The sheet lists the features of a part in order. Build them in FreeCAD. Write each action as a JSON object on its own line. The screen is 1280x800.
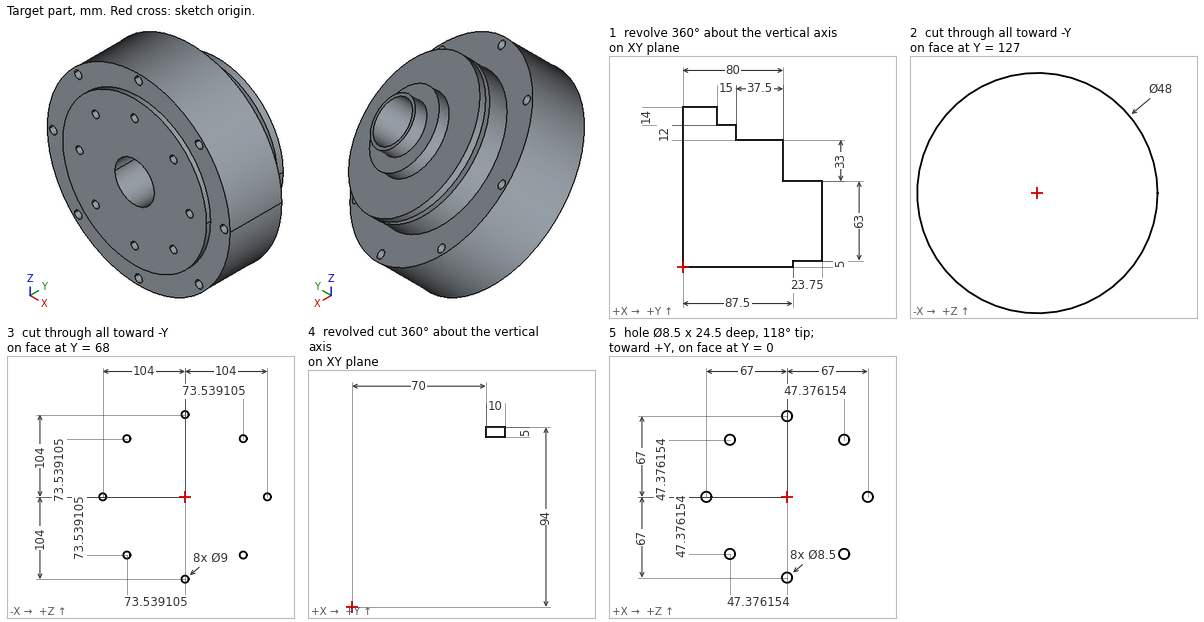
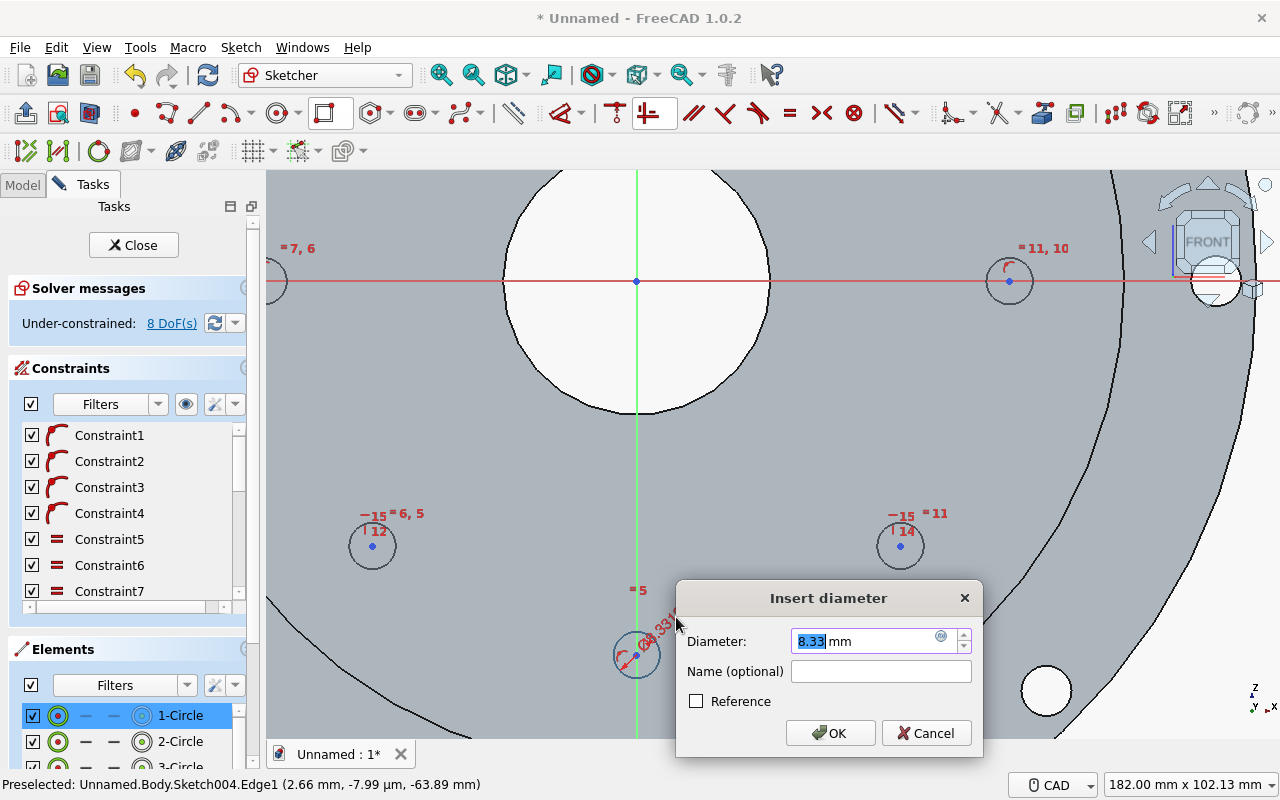
{"action": "type", "text": "8.5"}
{"action": "key", "text": "Return"}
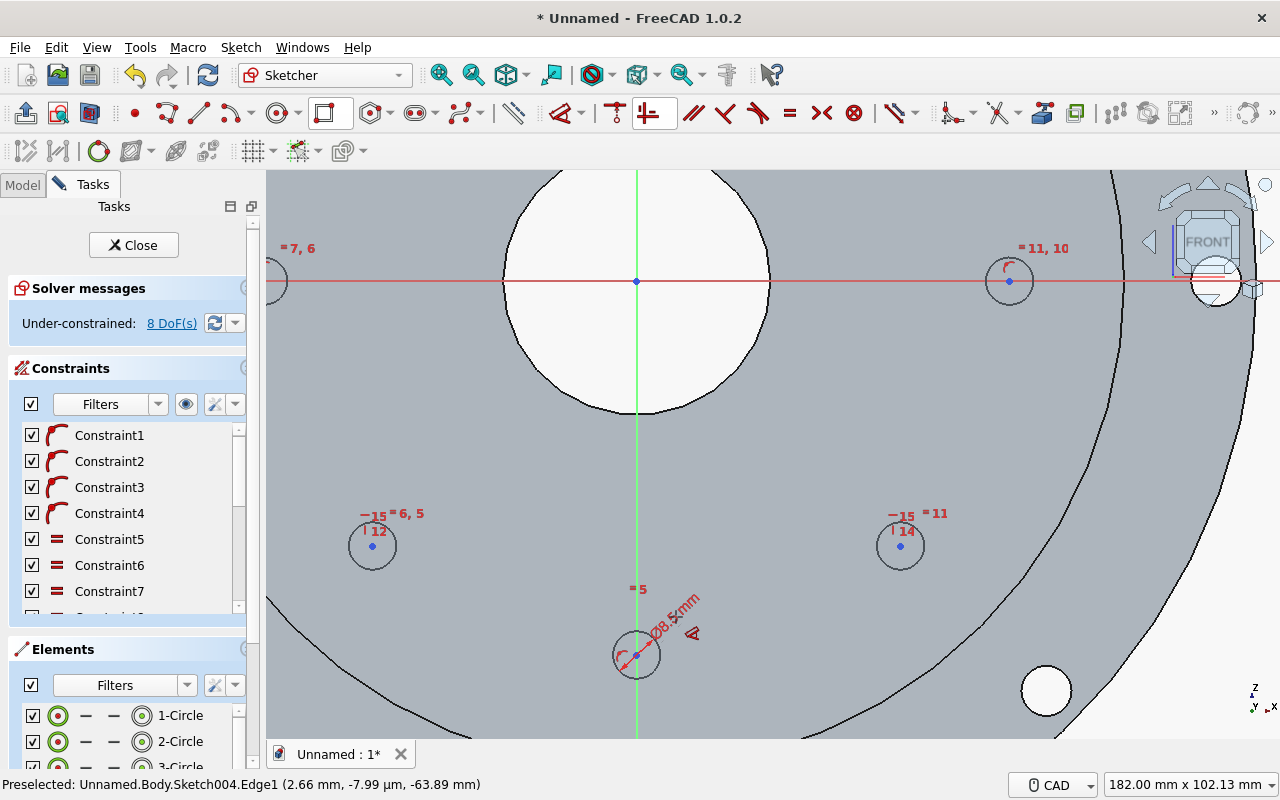
{"action": "left_click", "coordinate": [637, 655]}
{"action": "left_click", "coordinate": [671, 468]}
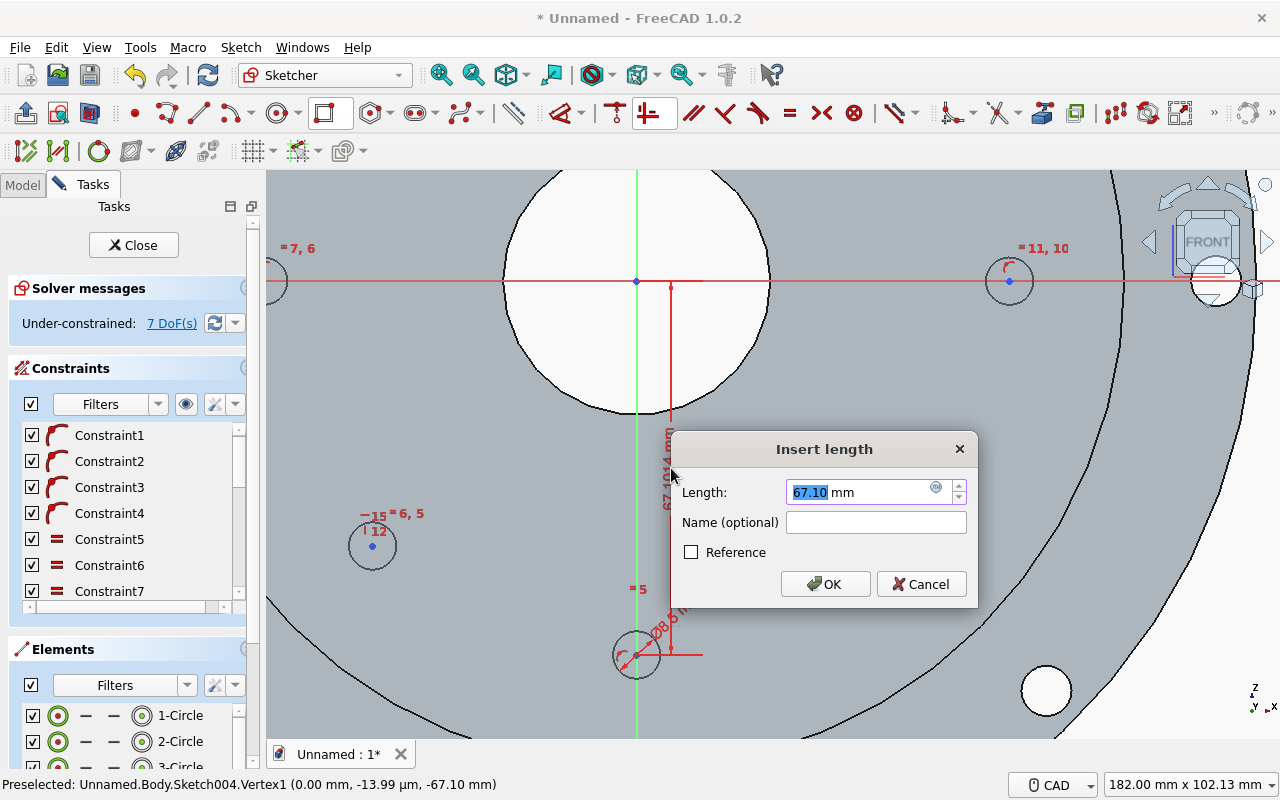
{"action": "type", "text": "67"}
{"action": "key", "text": "Return"}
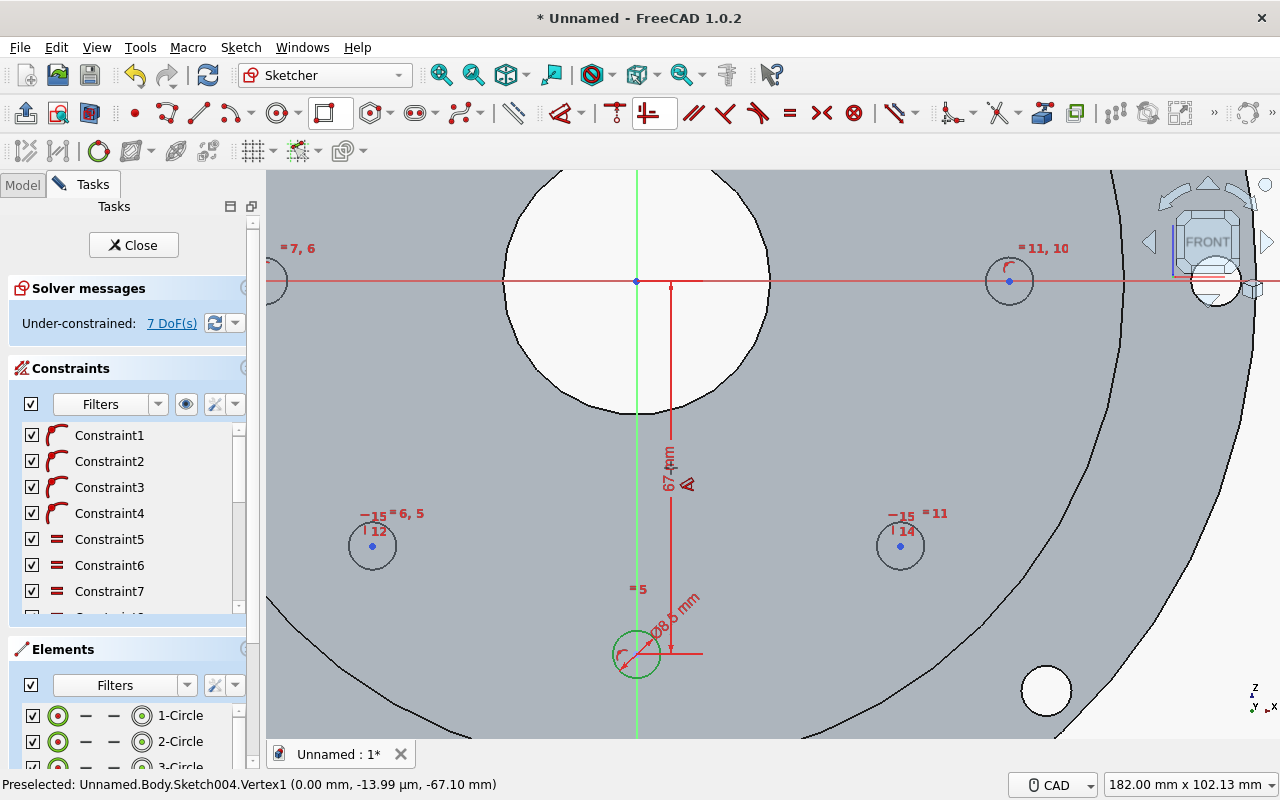
{"action": "scroll", "coordinate": [760, 596], "scroll_direction": "down", "scroll_amount": 4}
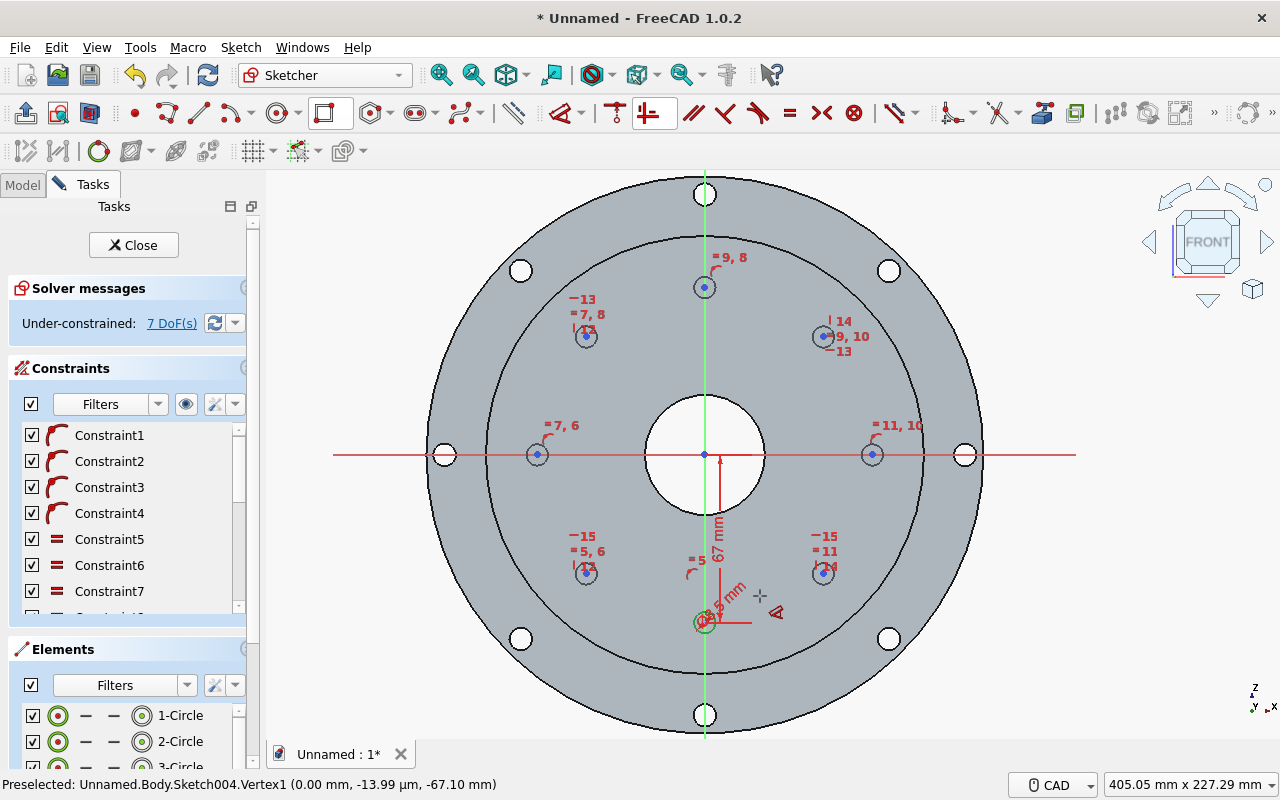
{"action": "left_click", "coordinate": [537, 455]}
{"action": "left_click", "coordinate": [621, 489]}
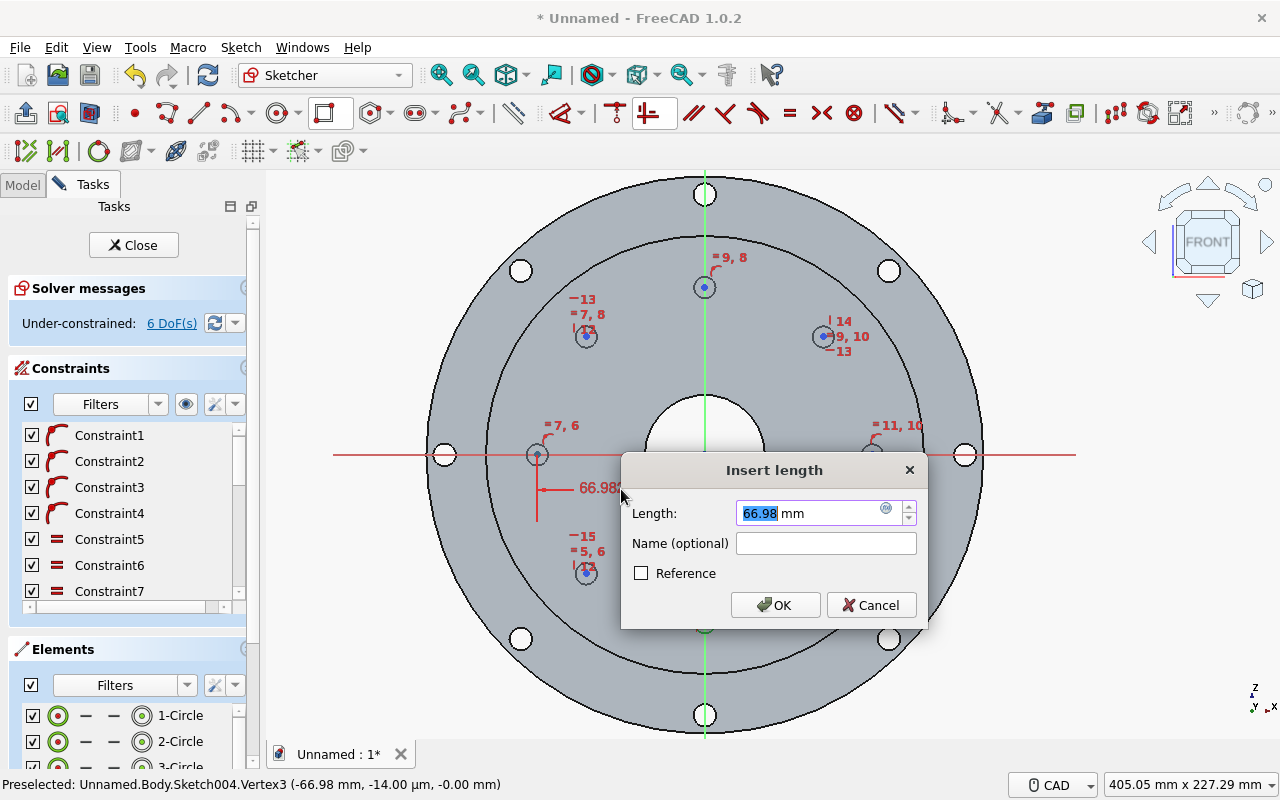
{"action": "type", "text": "67"}
{"action": "key", "text": "Return"}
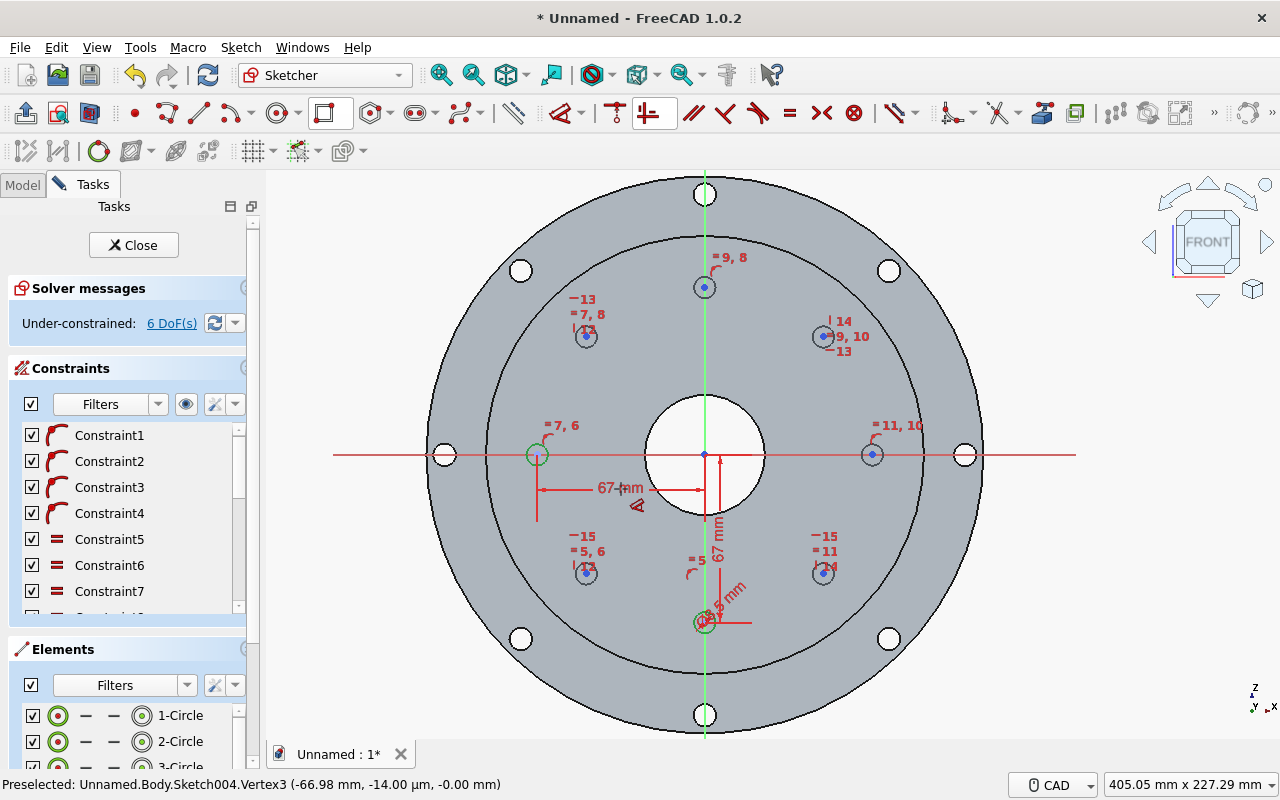
{"action": "left_click", "coordinate": [705, 288]}
{"action": "left_click", "coordinate": [739, 371]}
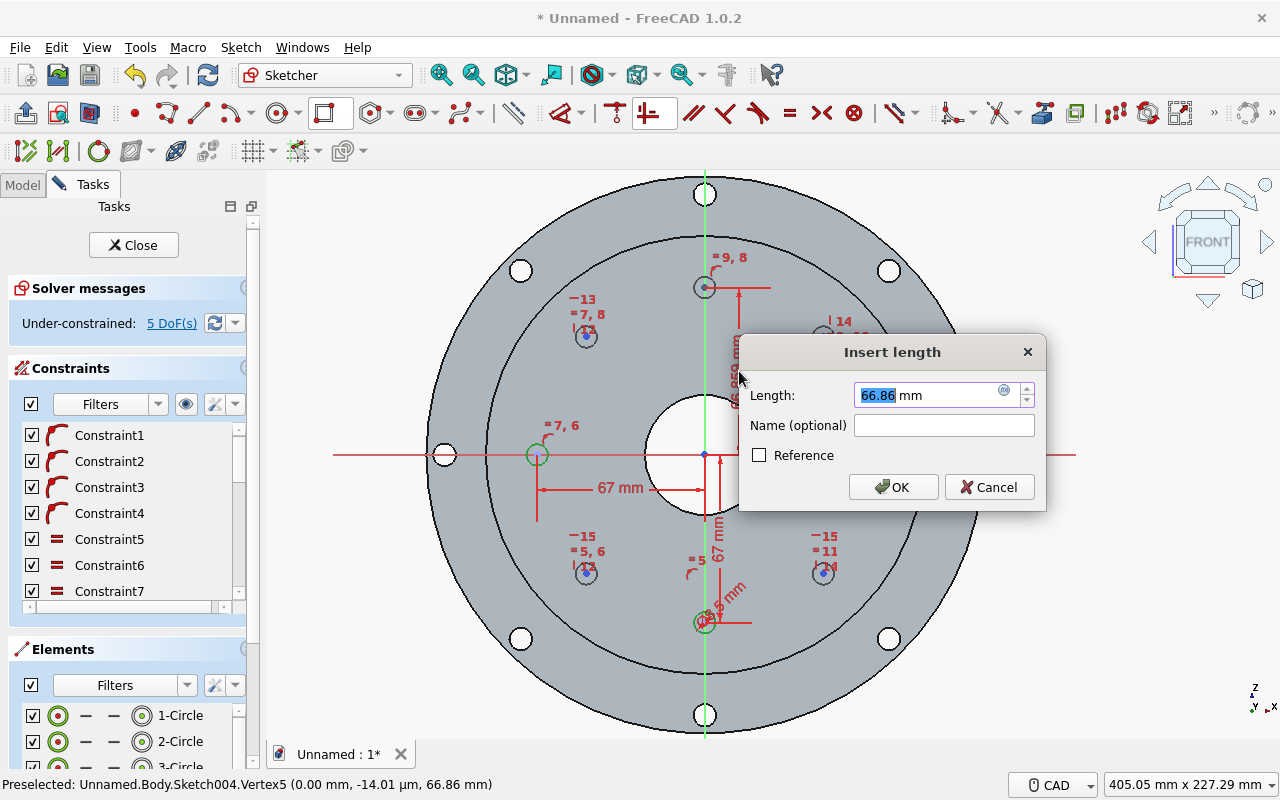
{"action": "type", "text": "67"}
{"action": "key", "text": "Return"}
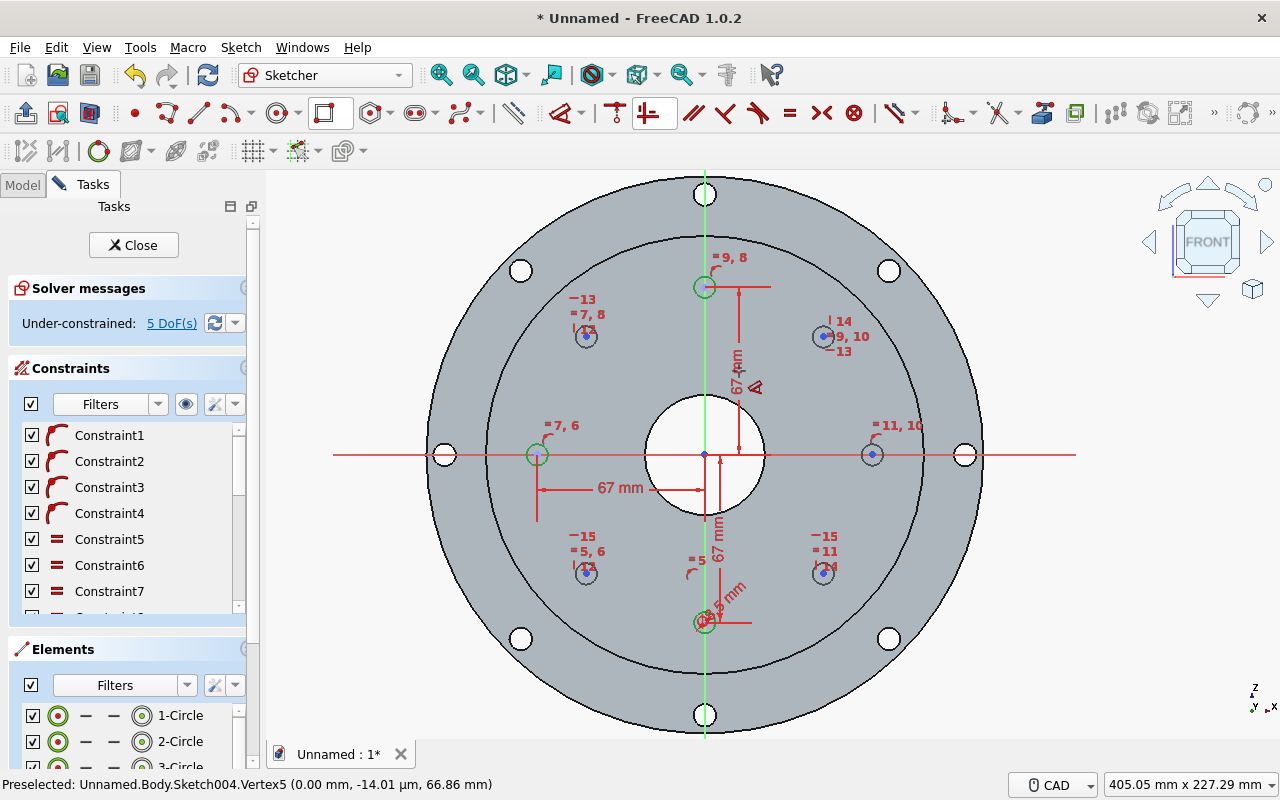
{"action": "left_click", "coordinate": [872, 455]}
{"action": "left_click", "coordinate": [789, 489]}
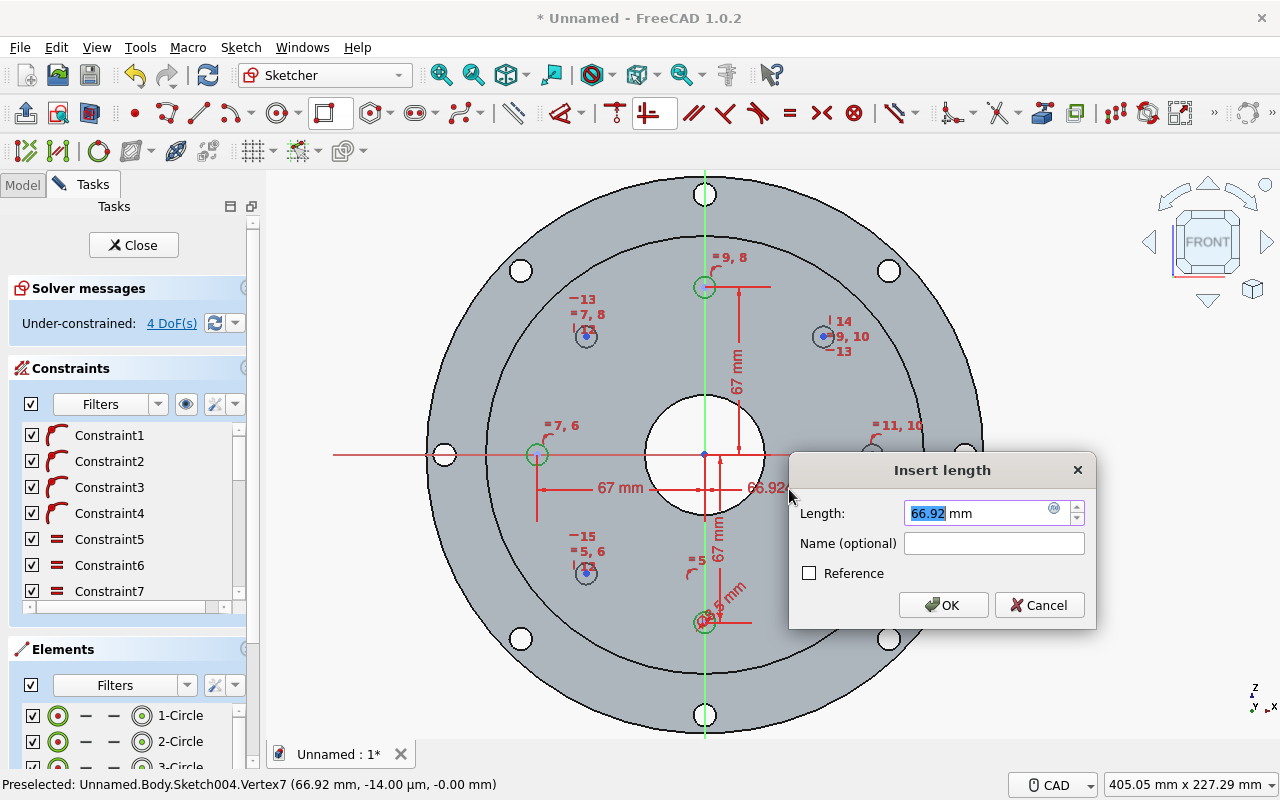
{"action": "type", "text": "67"}
{"action": "key", "text": "Return"}